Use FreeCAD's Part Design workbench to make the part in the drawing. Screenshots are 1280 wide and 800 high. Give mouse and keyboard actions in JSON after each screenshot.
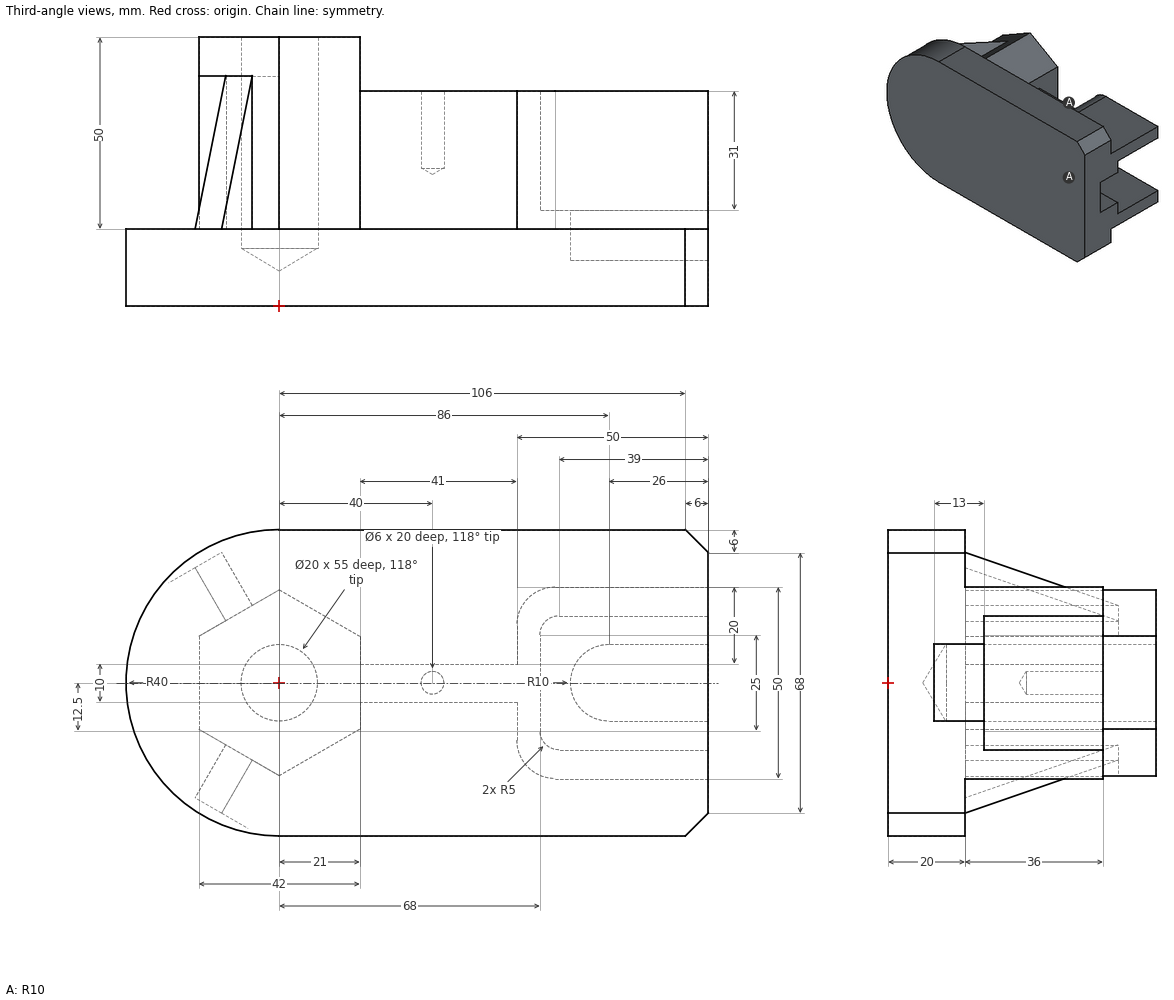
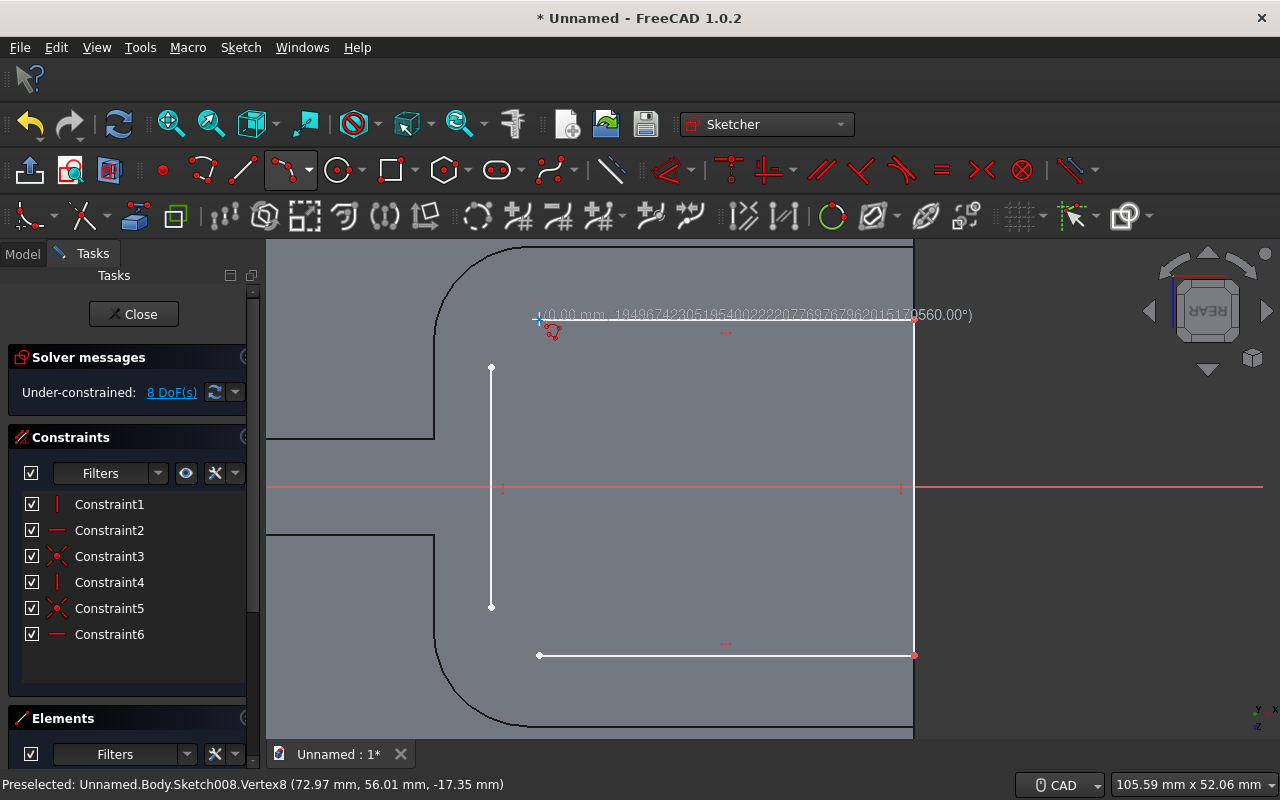
{"action": "left_click", "coordinate": [284, 170]}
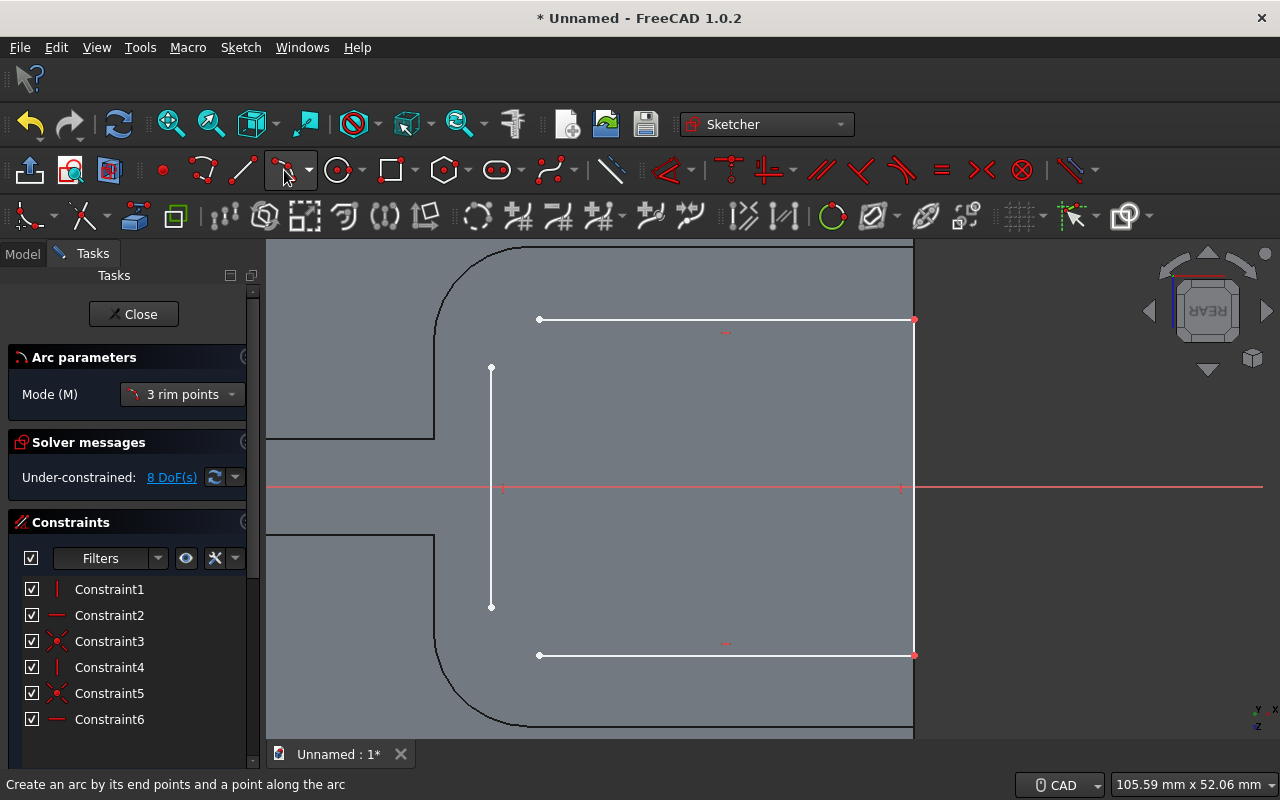
{"action": "left_click", "coordinate": [491, 608]}
{"action": "left_click", "coordinate": [539, 656]}
{"action": "left_click", "coordinate": [505, 641]}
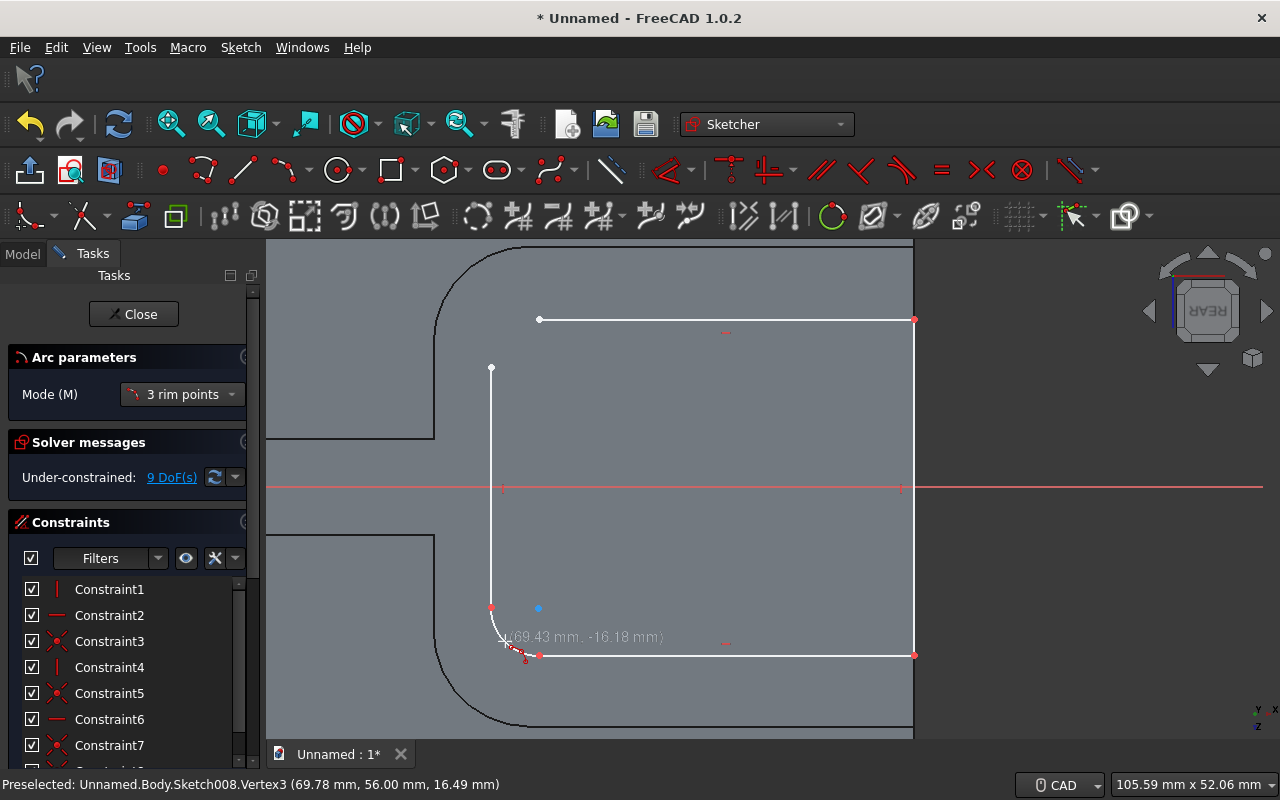
{"action": "left_click", "coordinate": [539, 320]}
{"action": "left_click", "coordinate": [491, 368]}
{"action": "left_click", "coordinate": [505, 333]}
{"action": "key", "text": "Escape"}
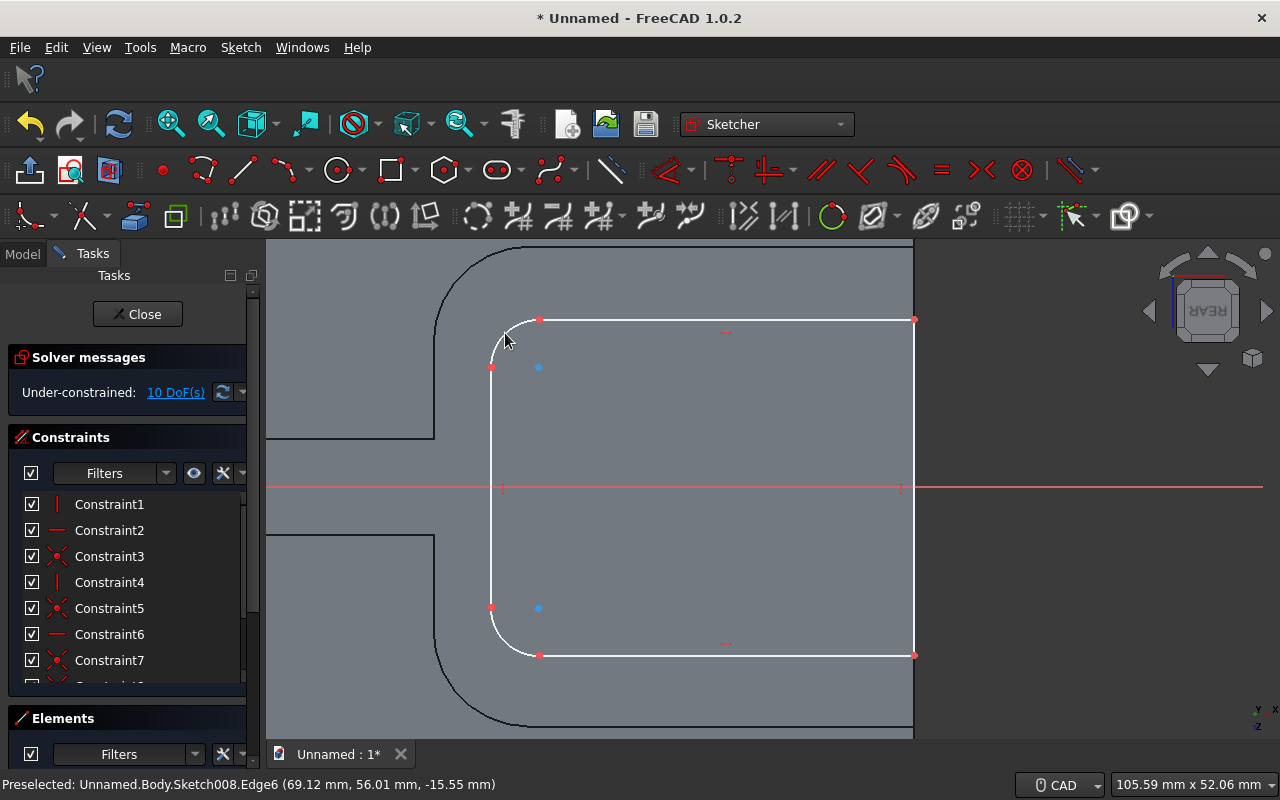
{"action": "left_click", "coordinate": [491, 440]}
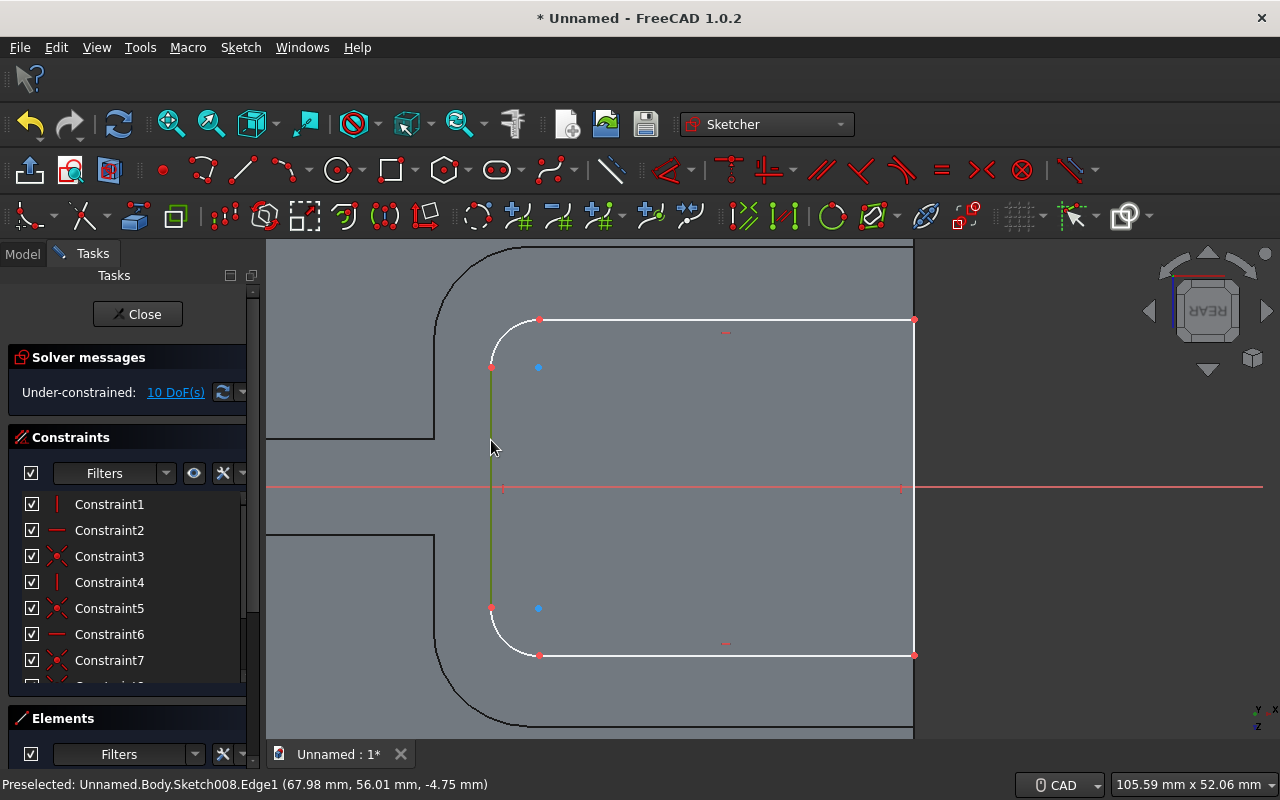
{"action": "left_click", "coordinate": [496, 630]}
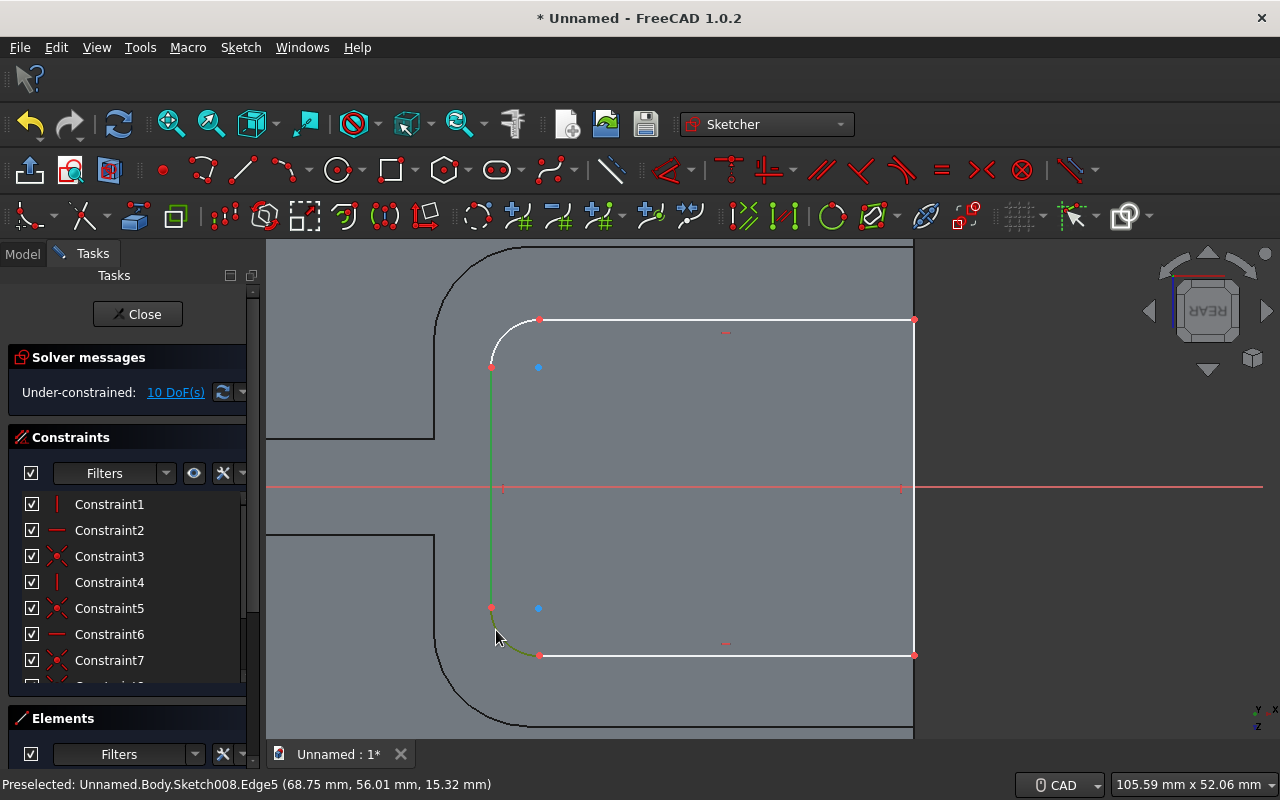
{"action": "left_click", "coordinate": [902, 170]}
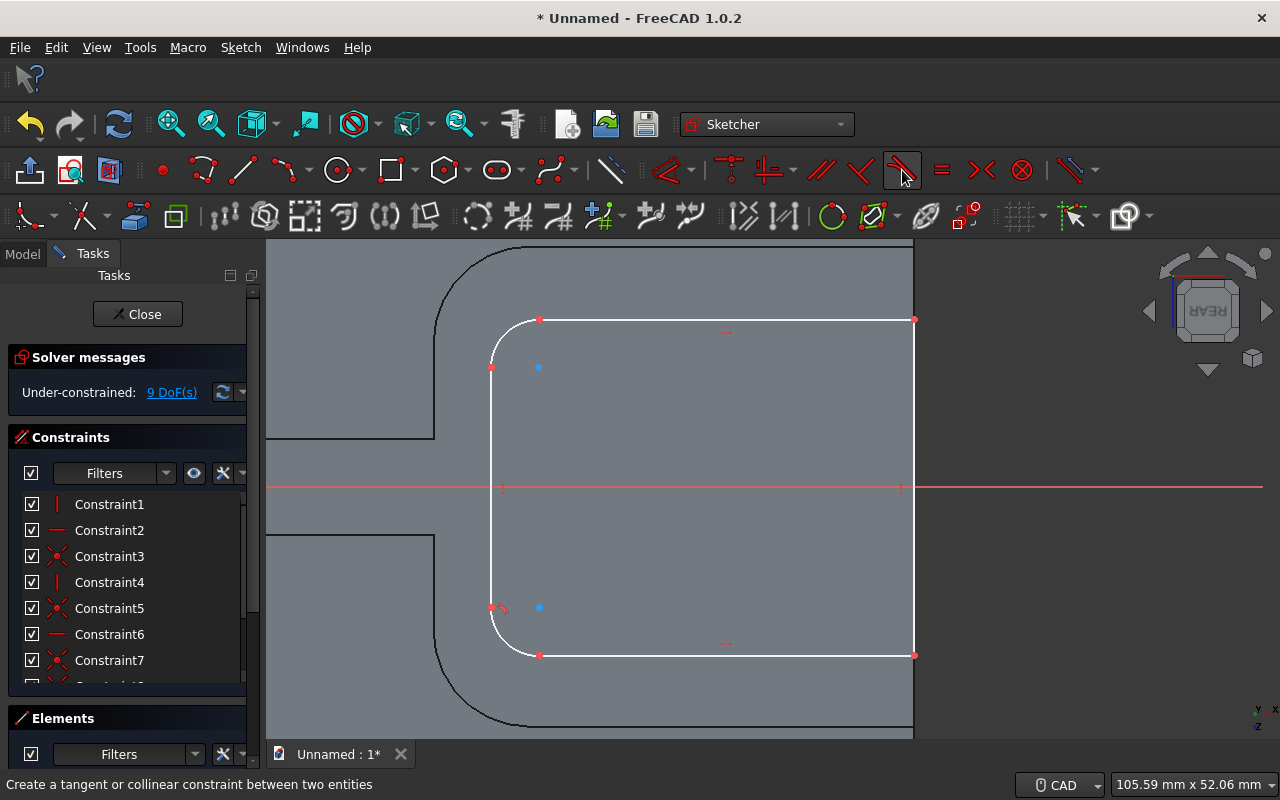
{"action": "left_click", "coordinate": [491, 440]}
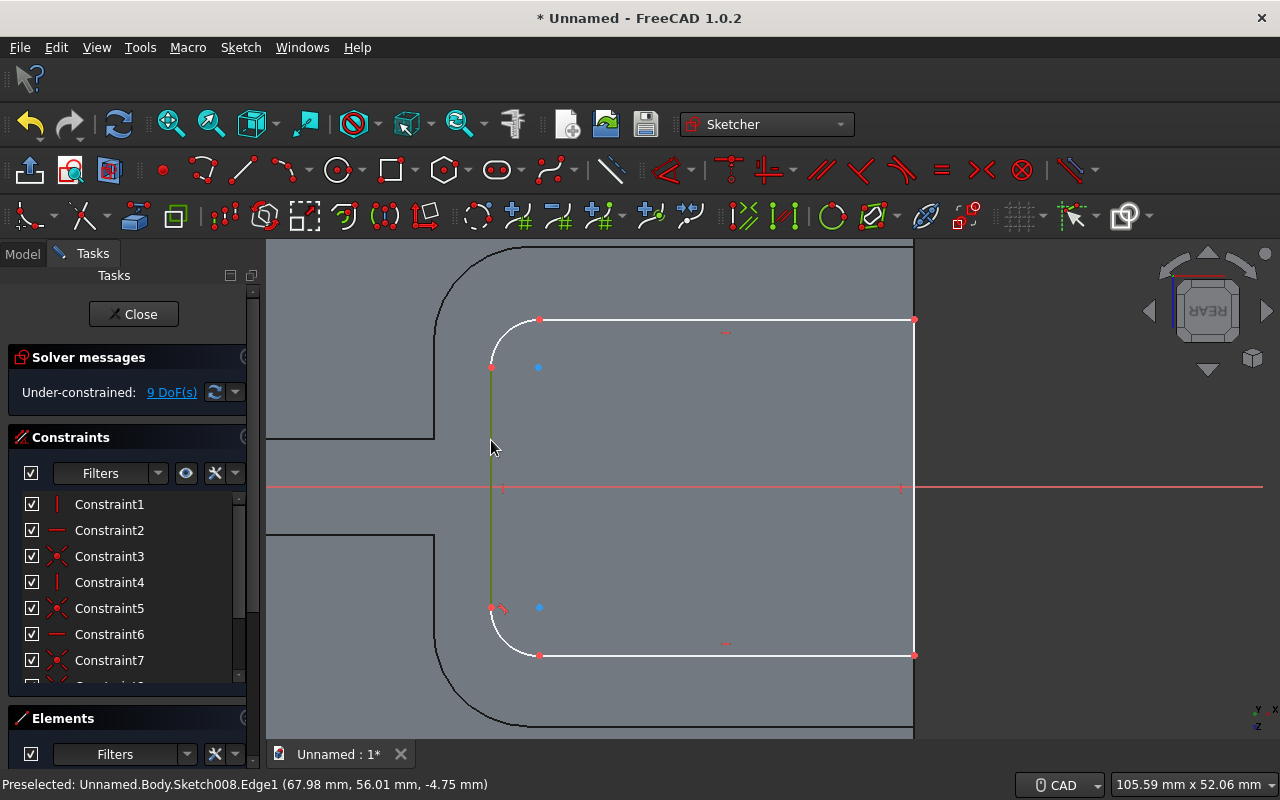
{"action": "left_click", "coordinate": [517, 325]}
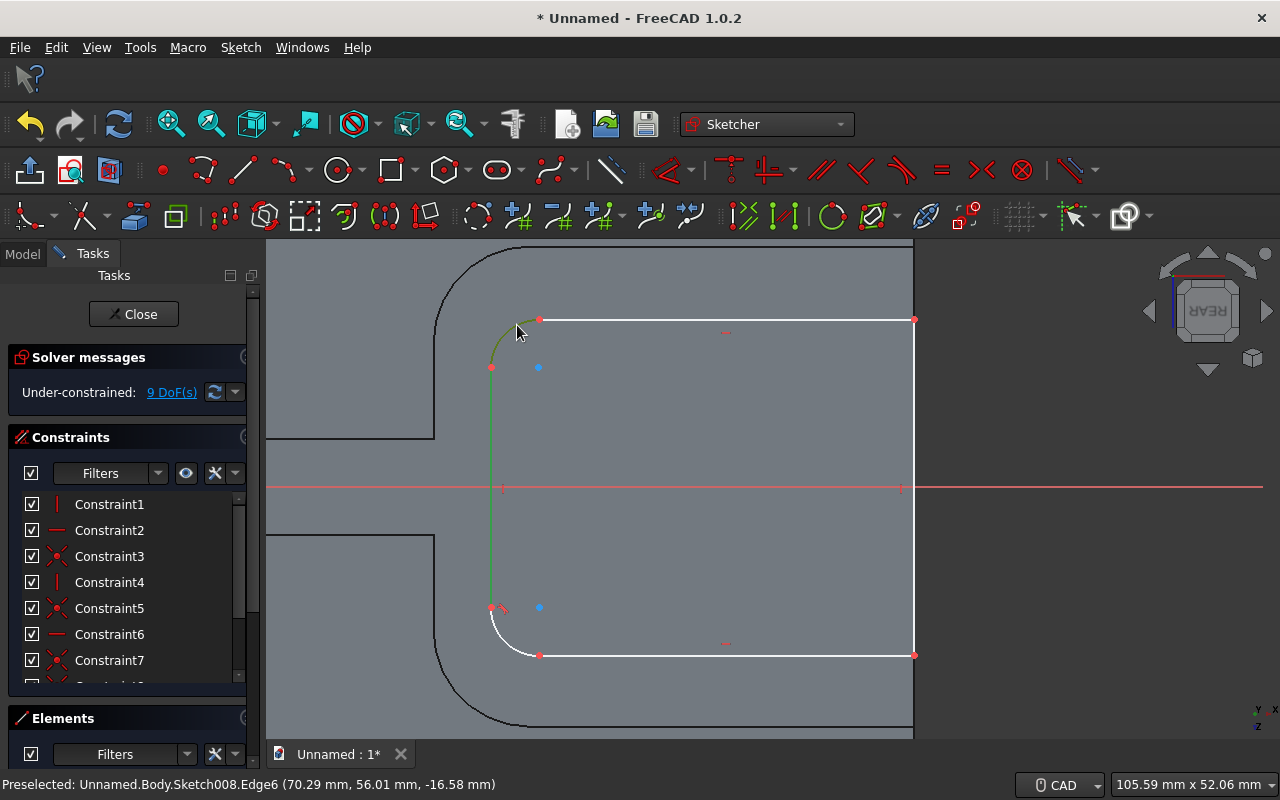
{"action": "left_click", "coordinate": [902, 170]}